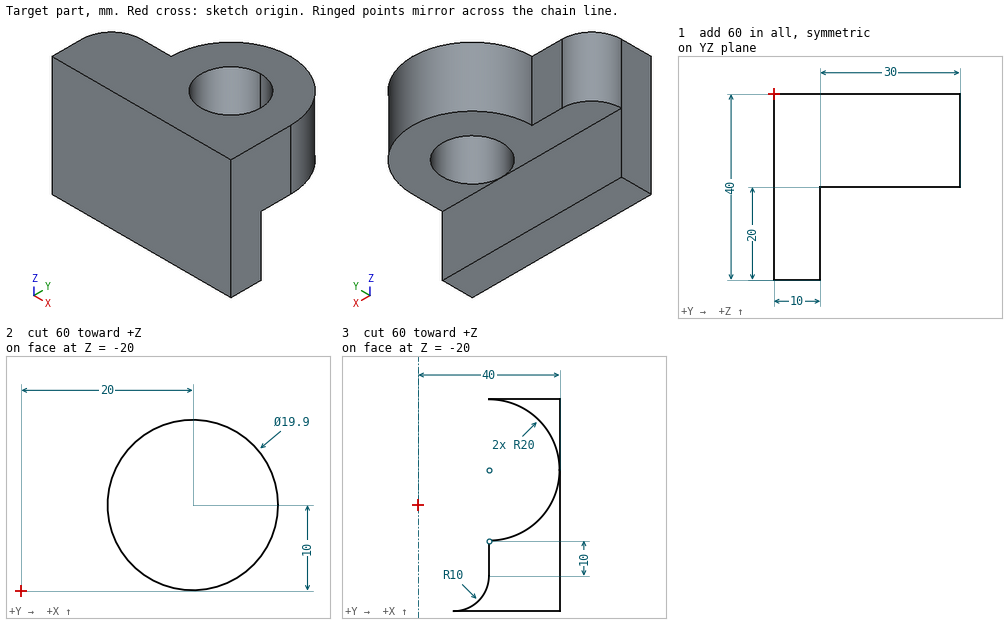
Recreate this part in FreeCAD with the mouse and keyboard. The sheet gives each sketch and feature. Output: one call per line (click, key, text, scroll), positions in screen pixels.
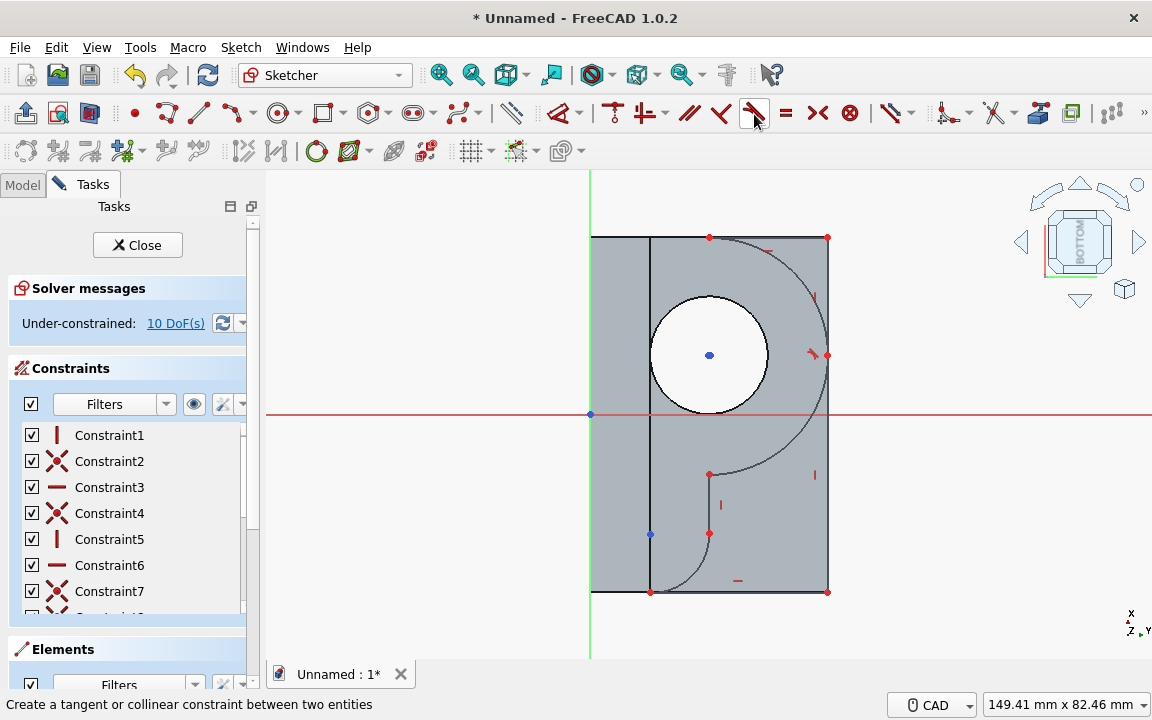
click(792, 238)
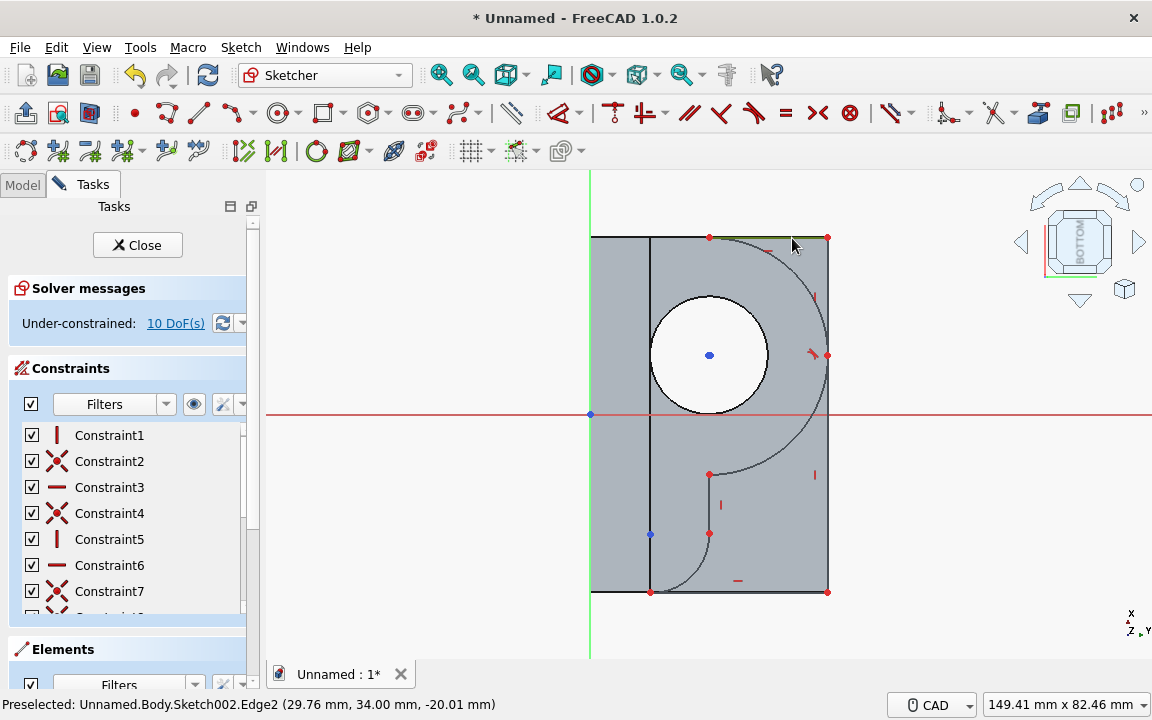
click(815, 302)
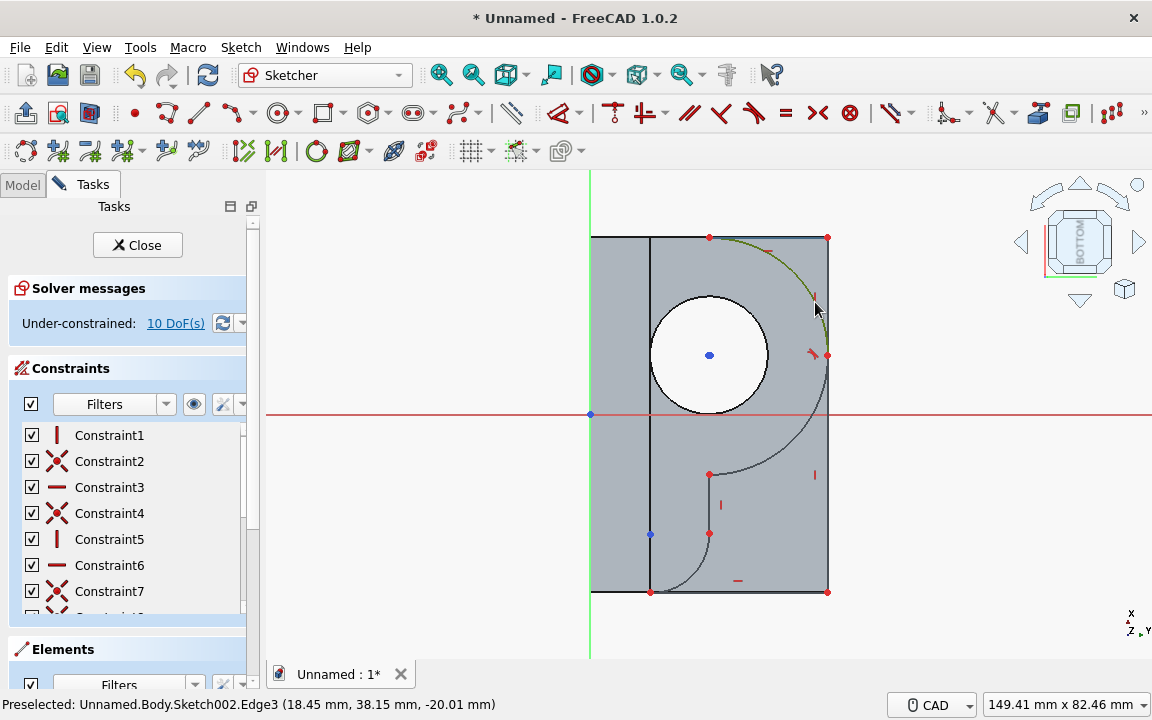
click(754, 114)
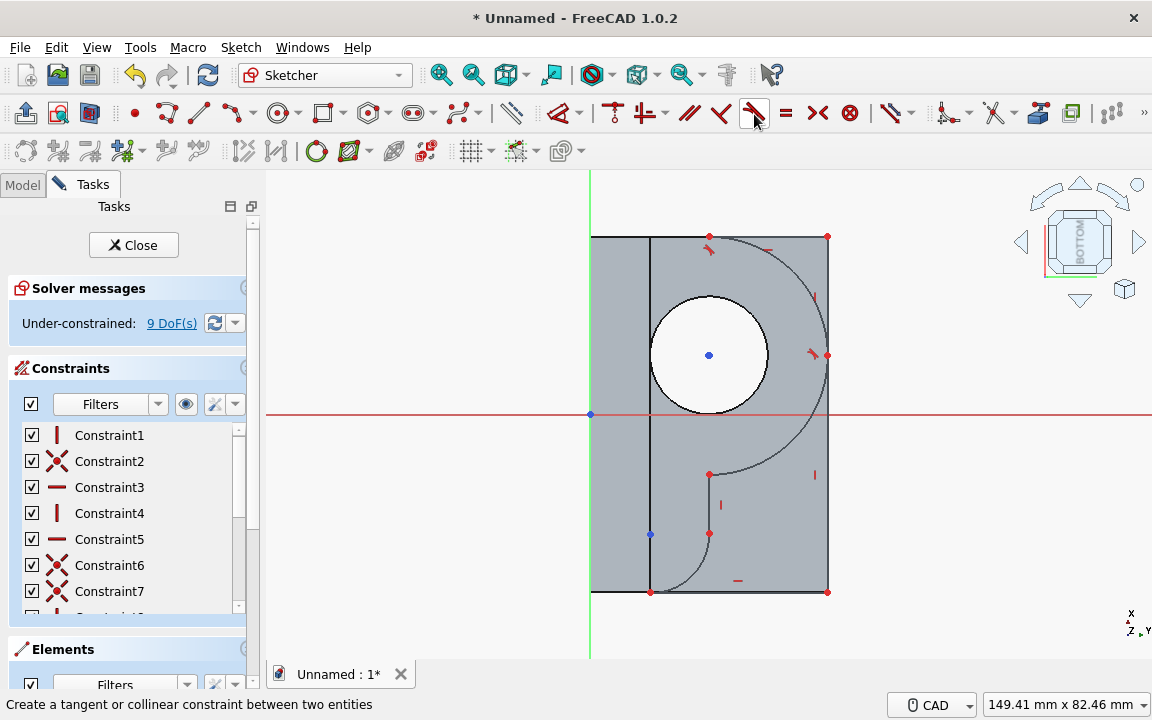
click(709, 493)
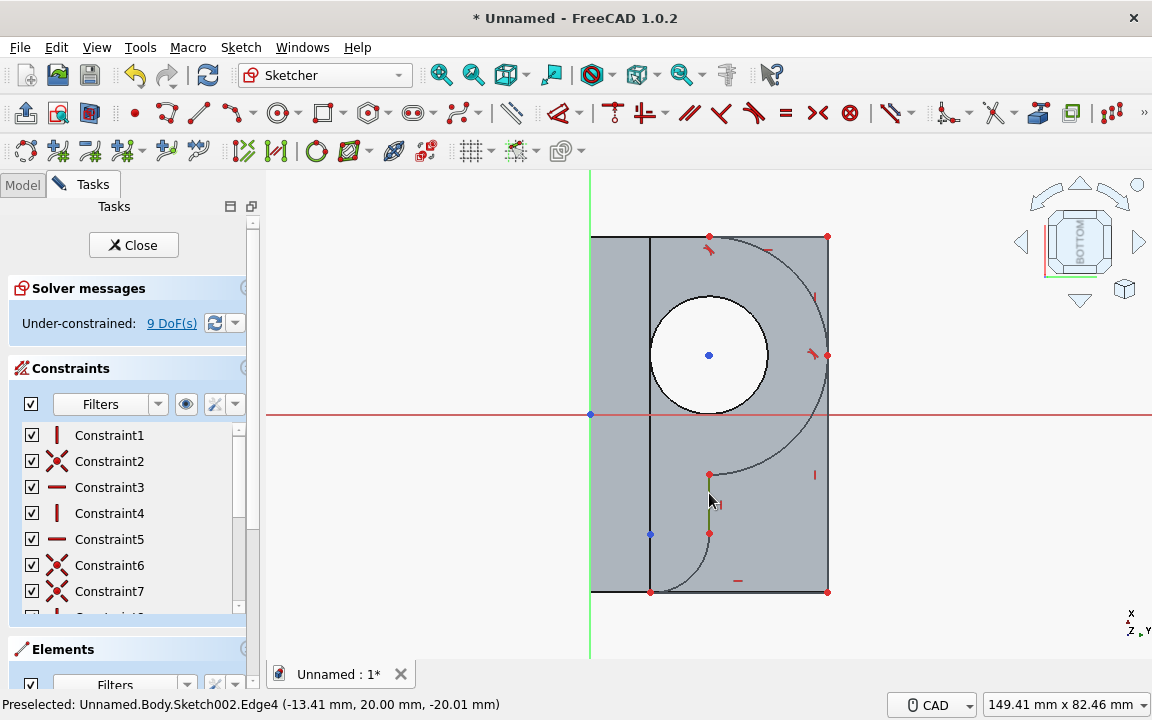
click(703, 561)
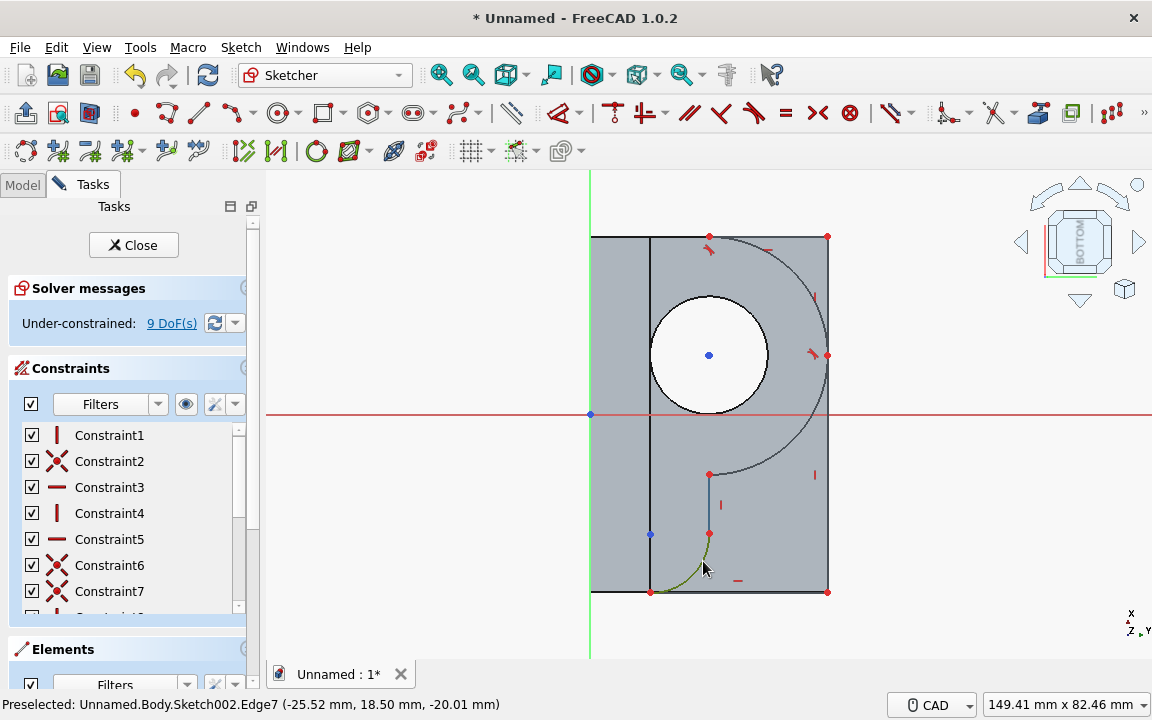
click(754, 114)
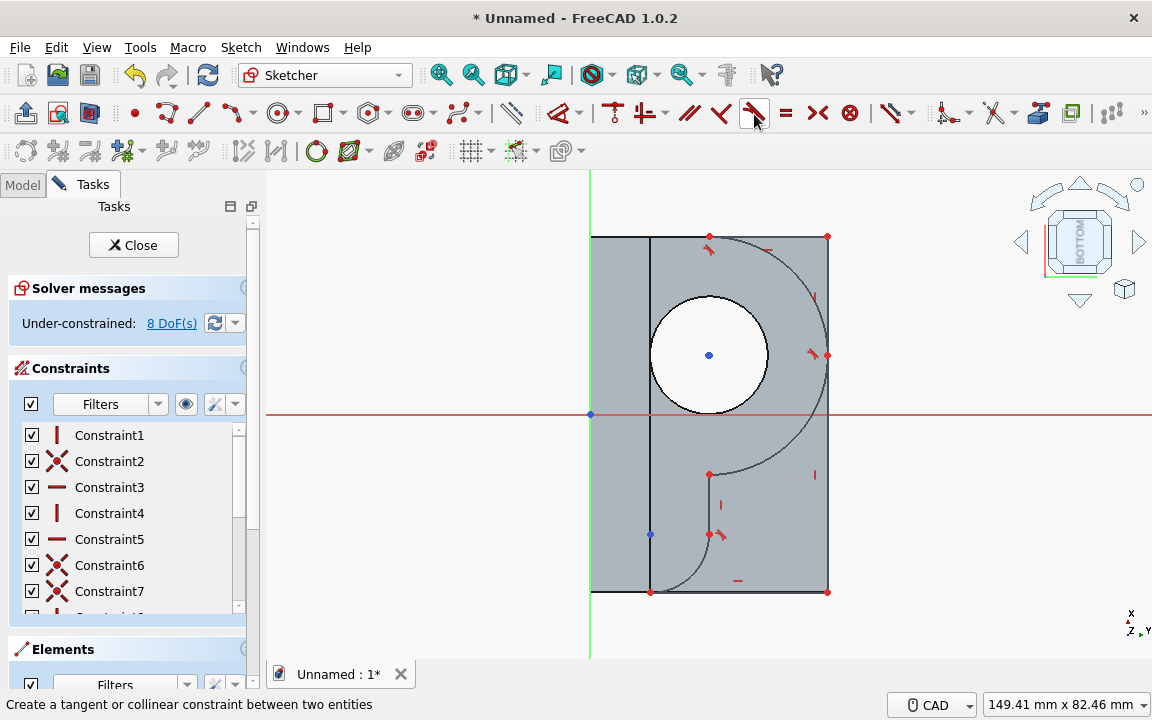
click(703, 593)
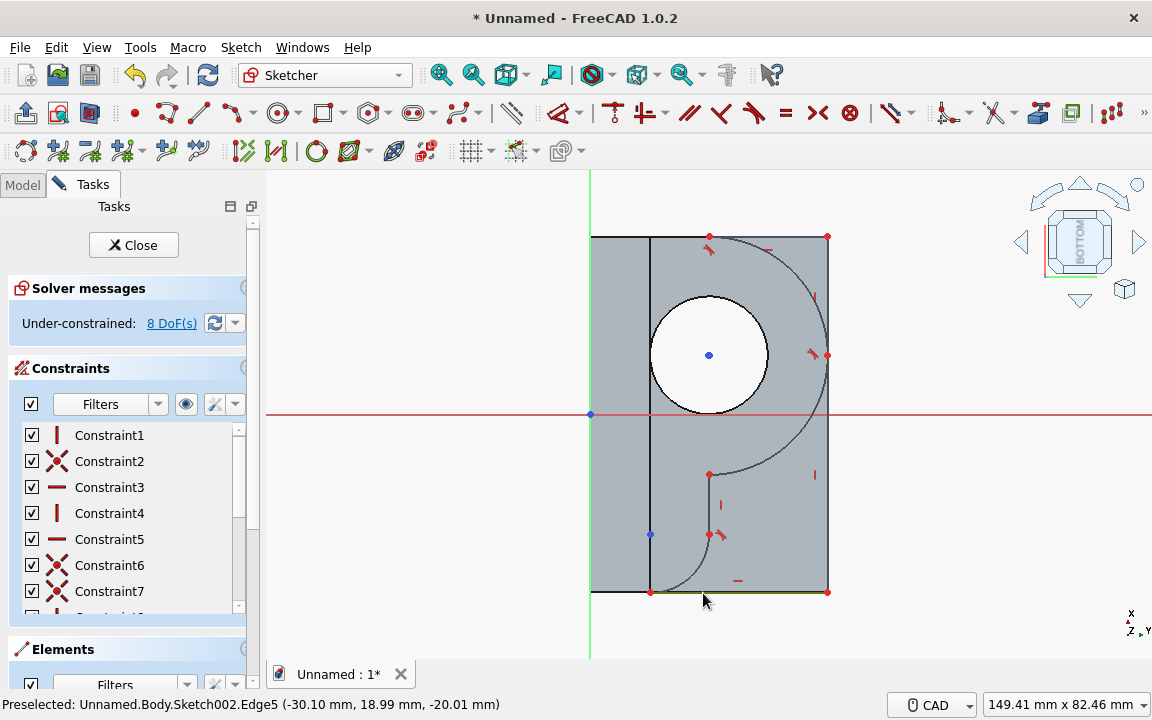
click(703, 561)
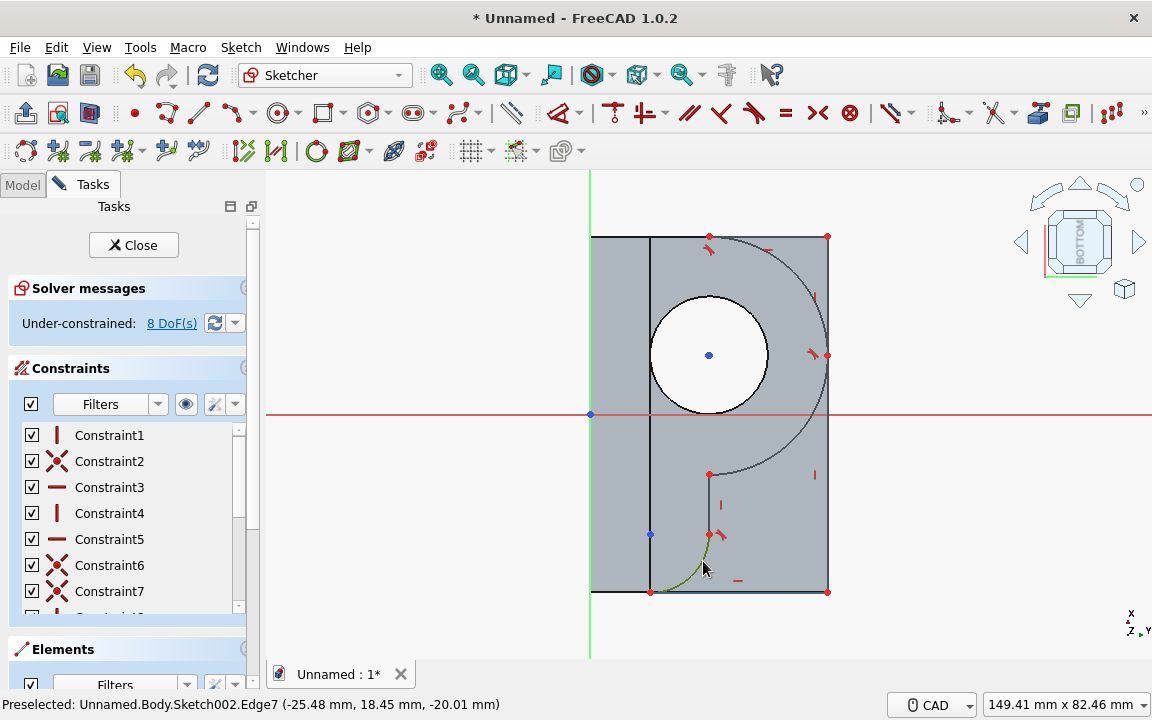
click(754, 114)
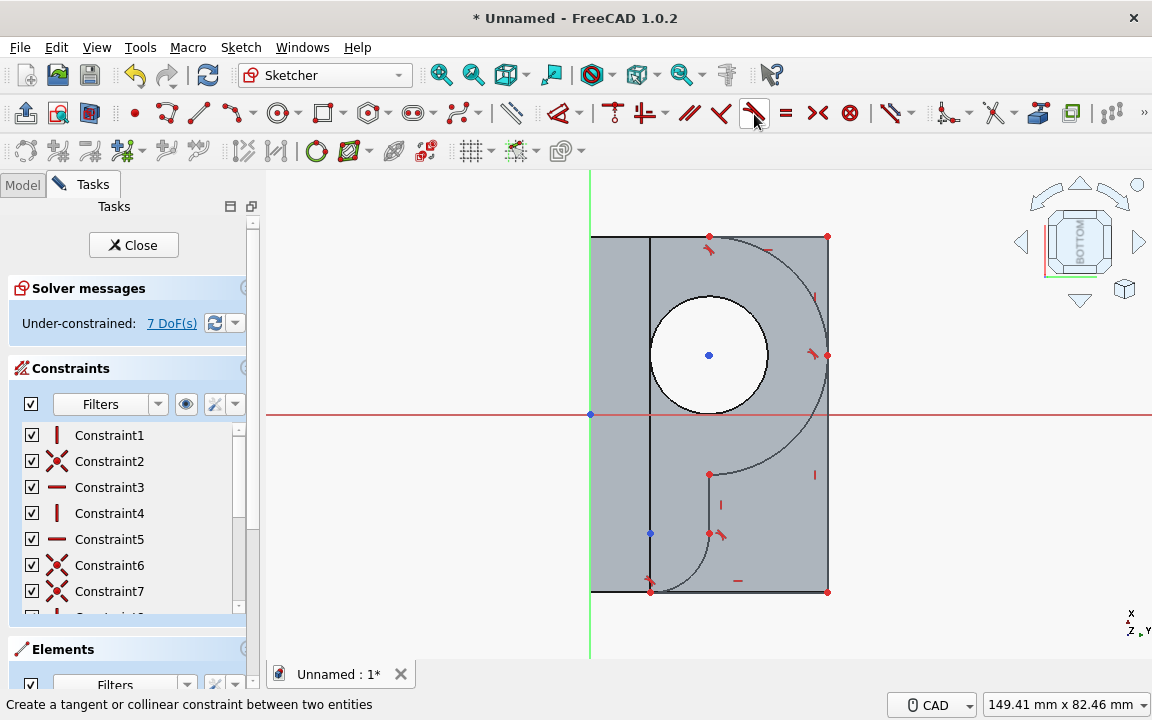
click(815, 302)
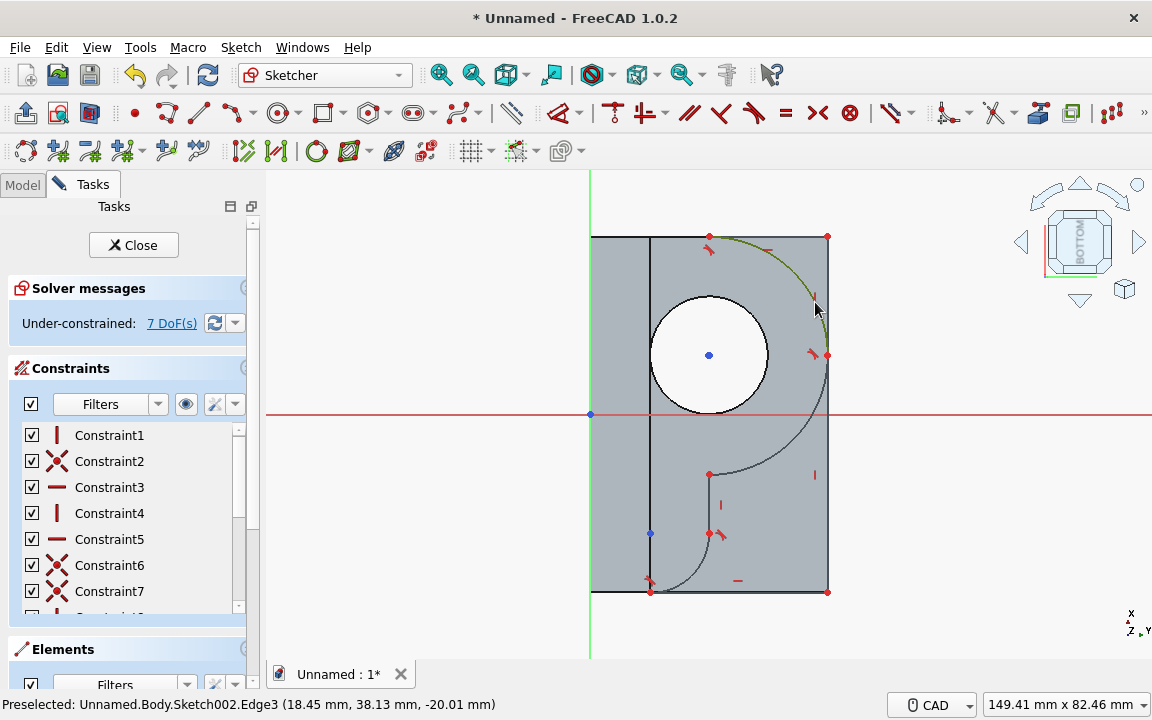
click(763, 462)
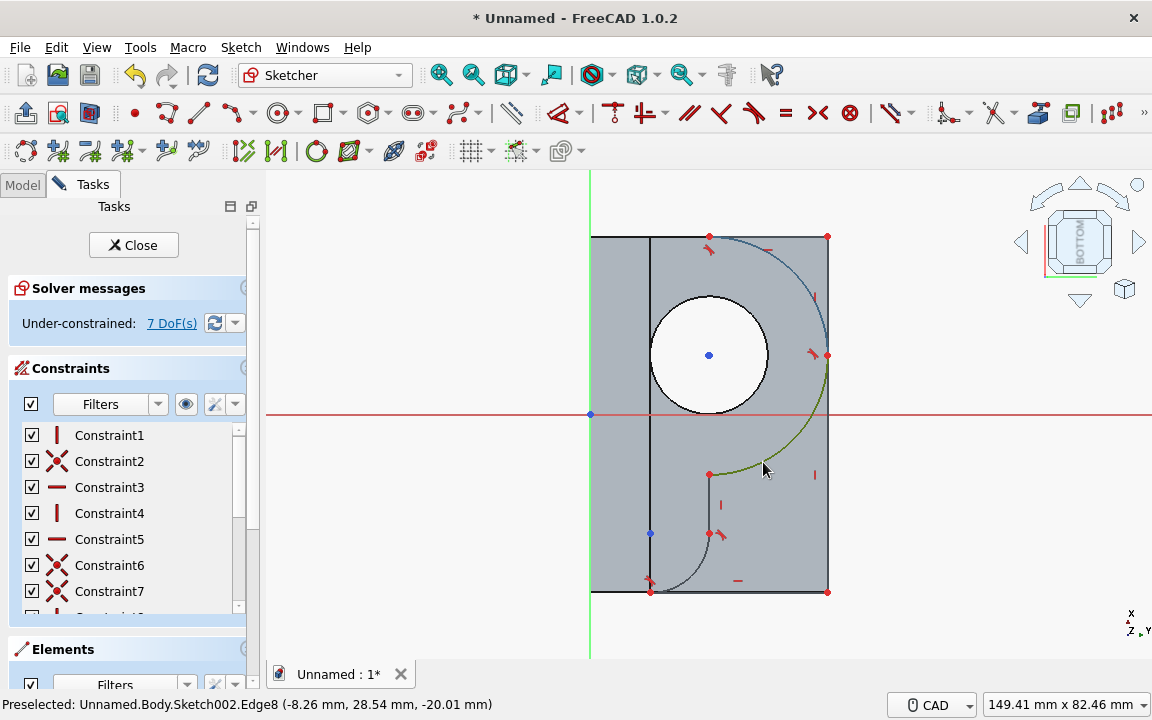
click(786, 114)